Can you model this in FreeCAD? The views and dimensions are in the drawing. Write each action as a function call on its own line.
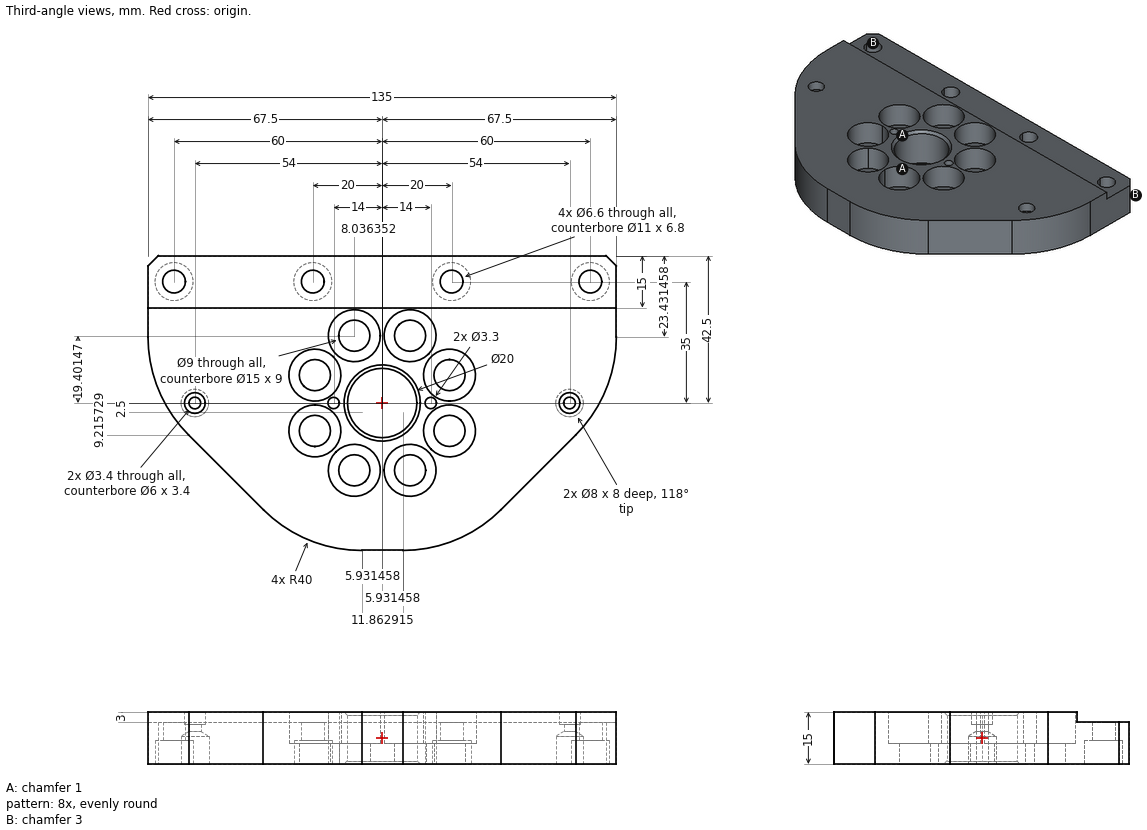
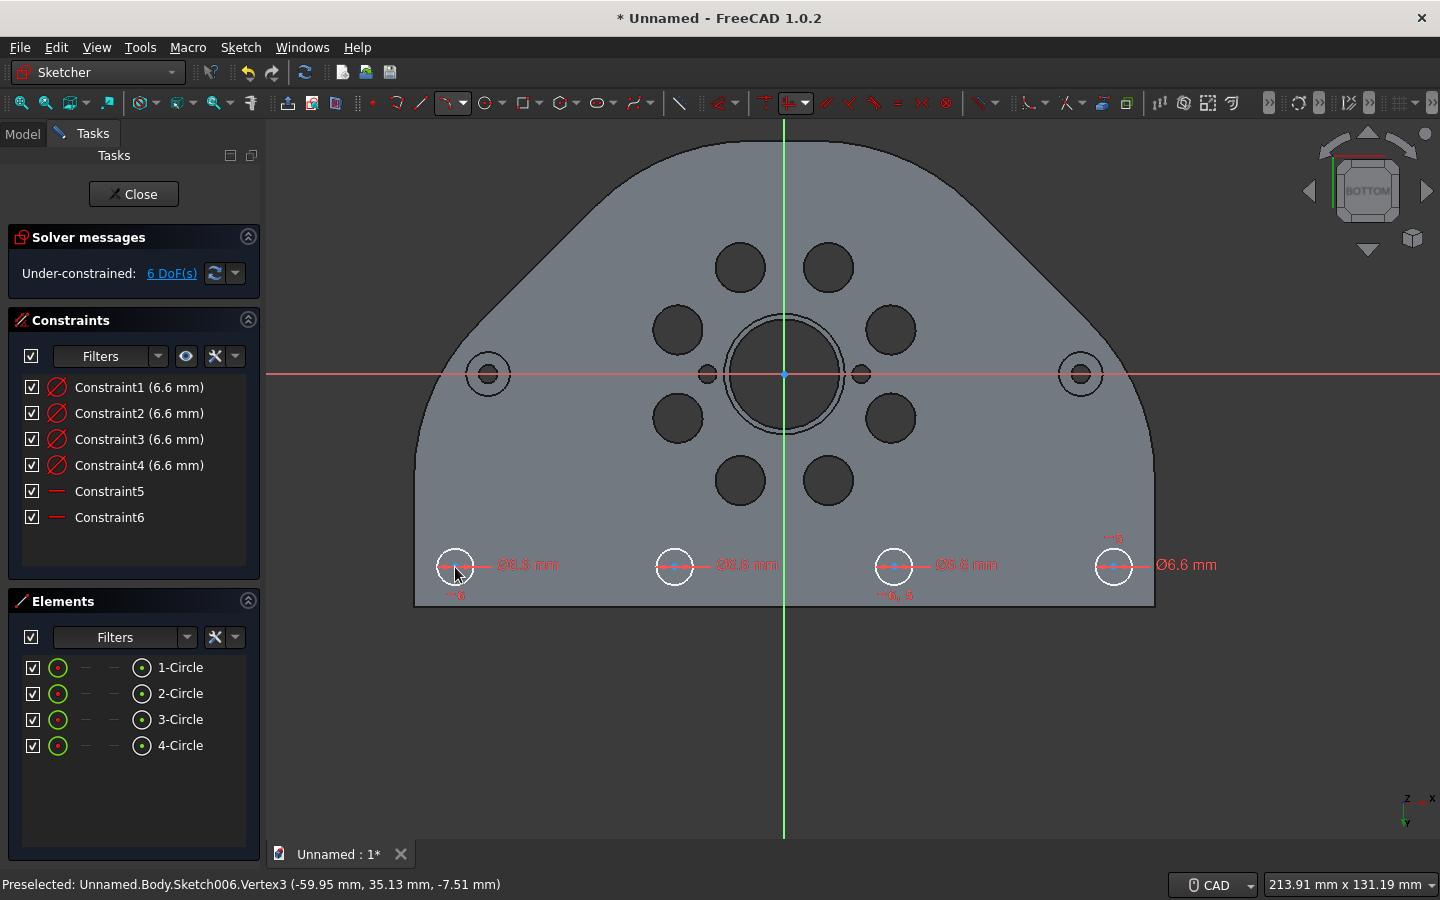
click(894, 567)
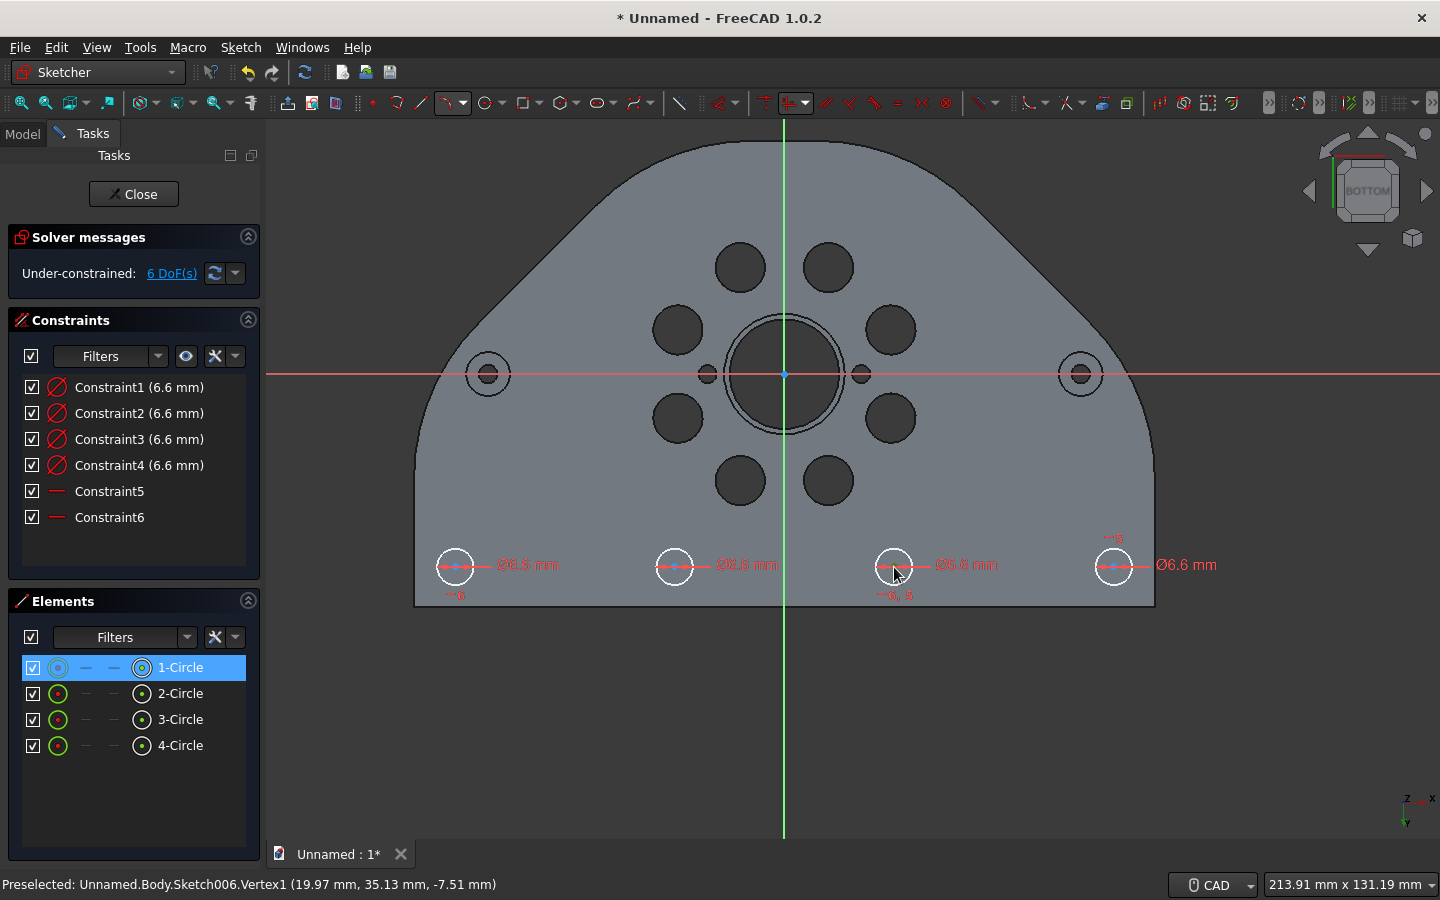
click(675, 567)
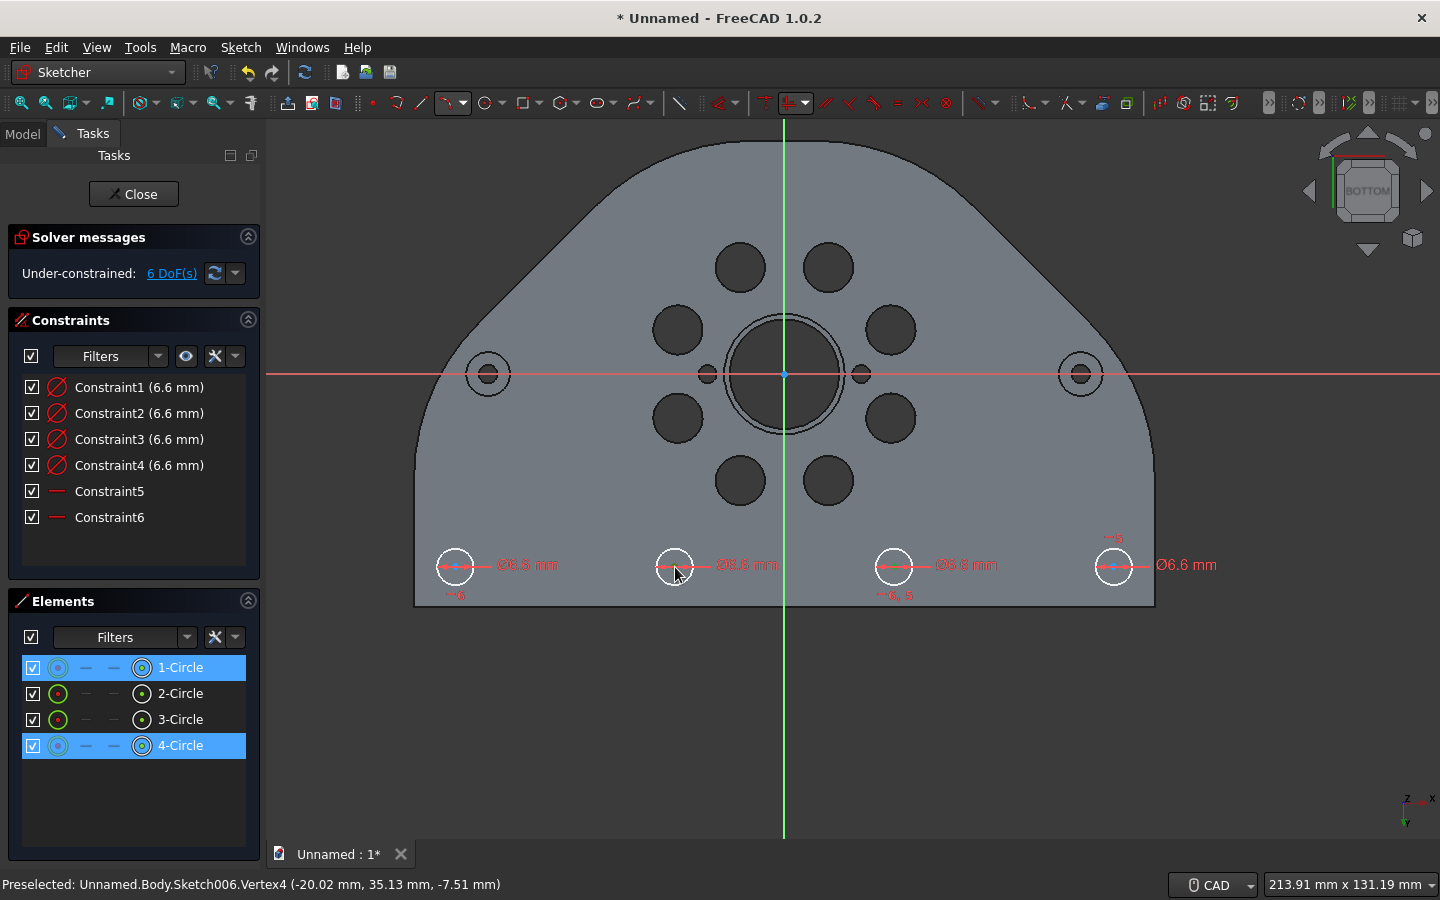
click(808, 104)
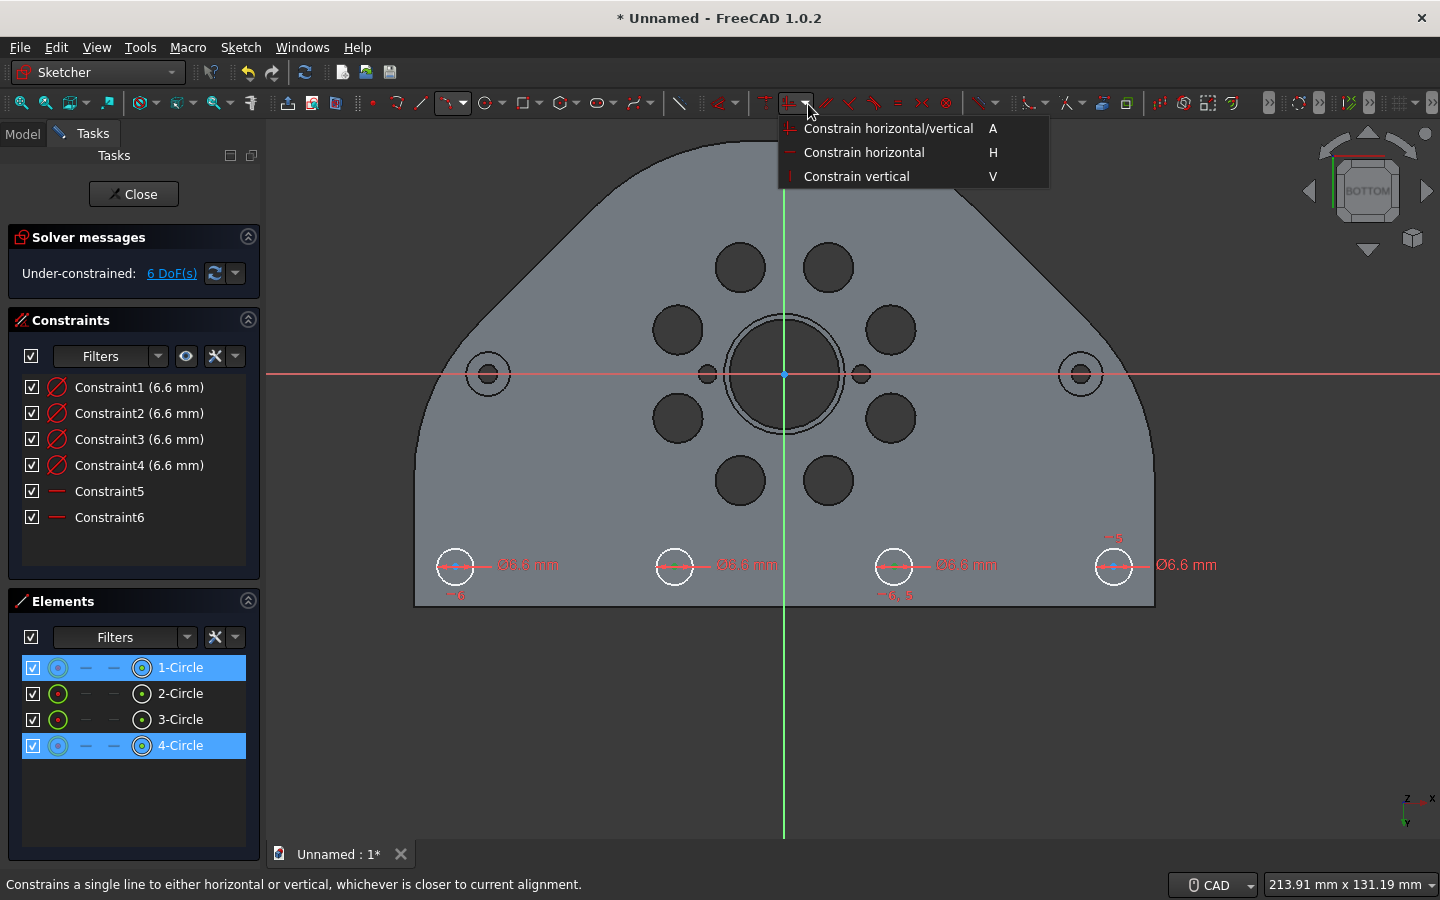
click(914, 152)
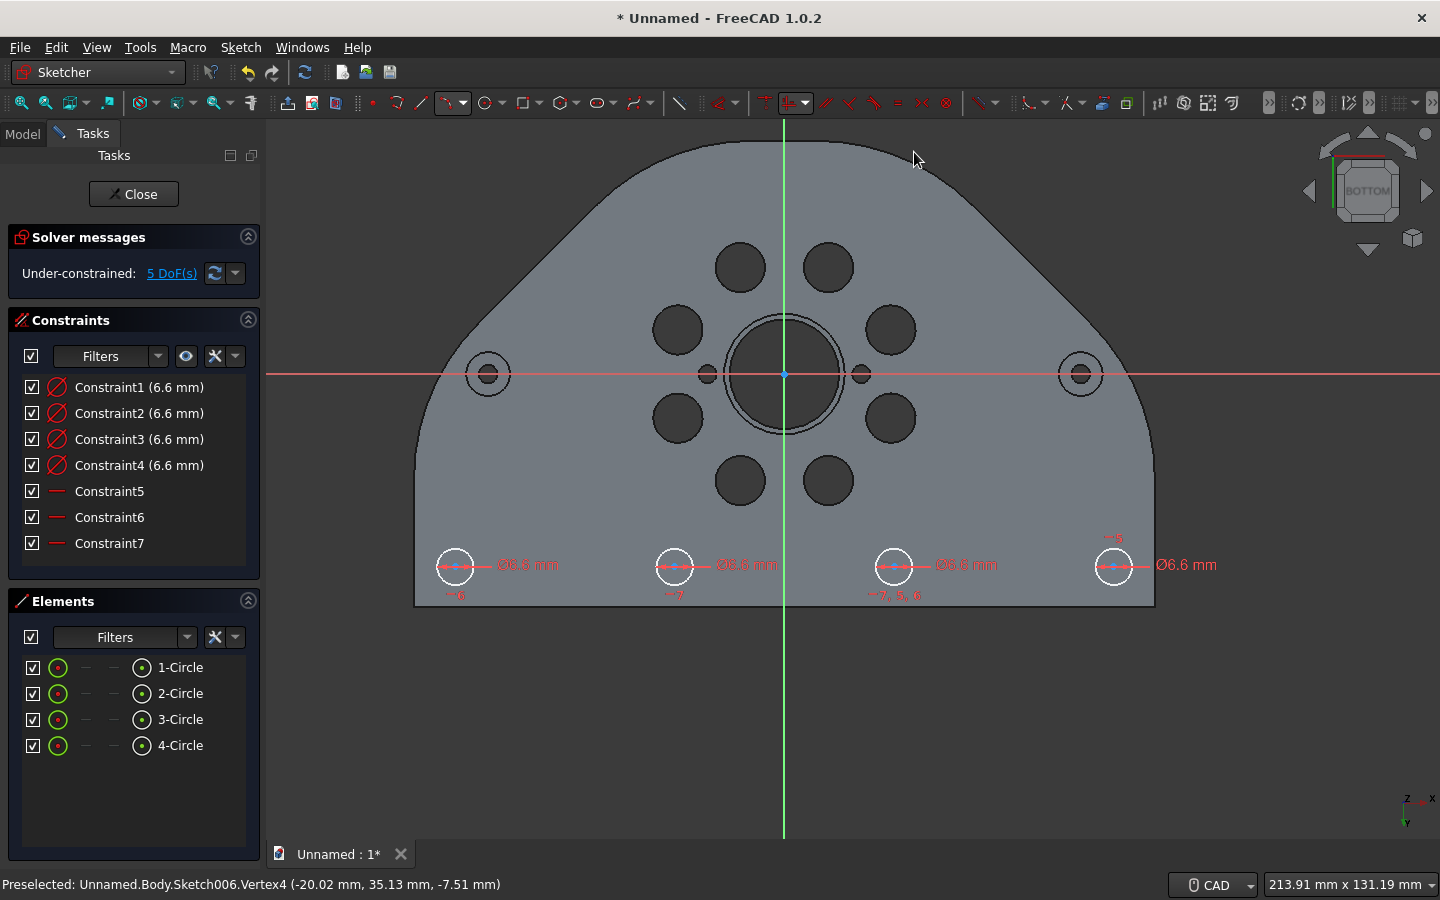
key(d)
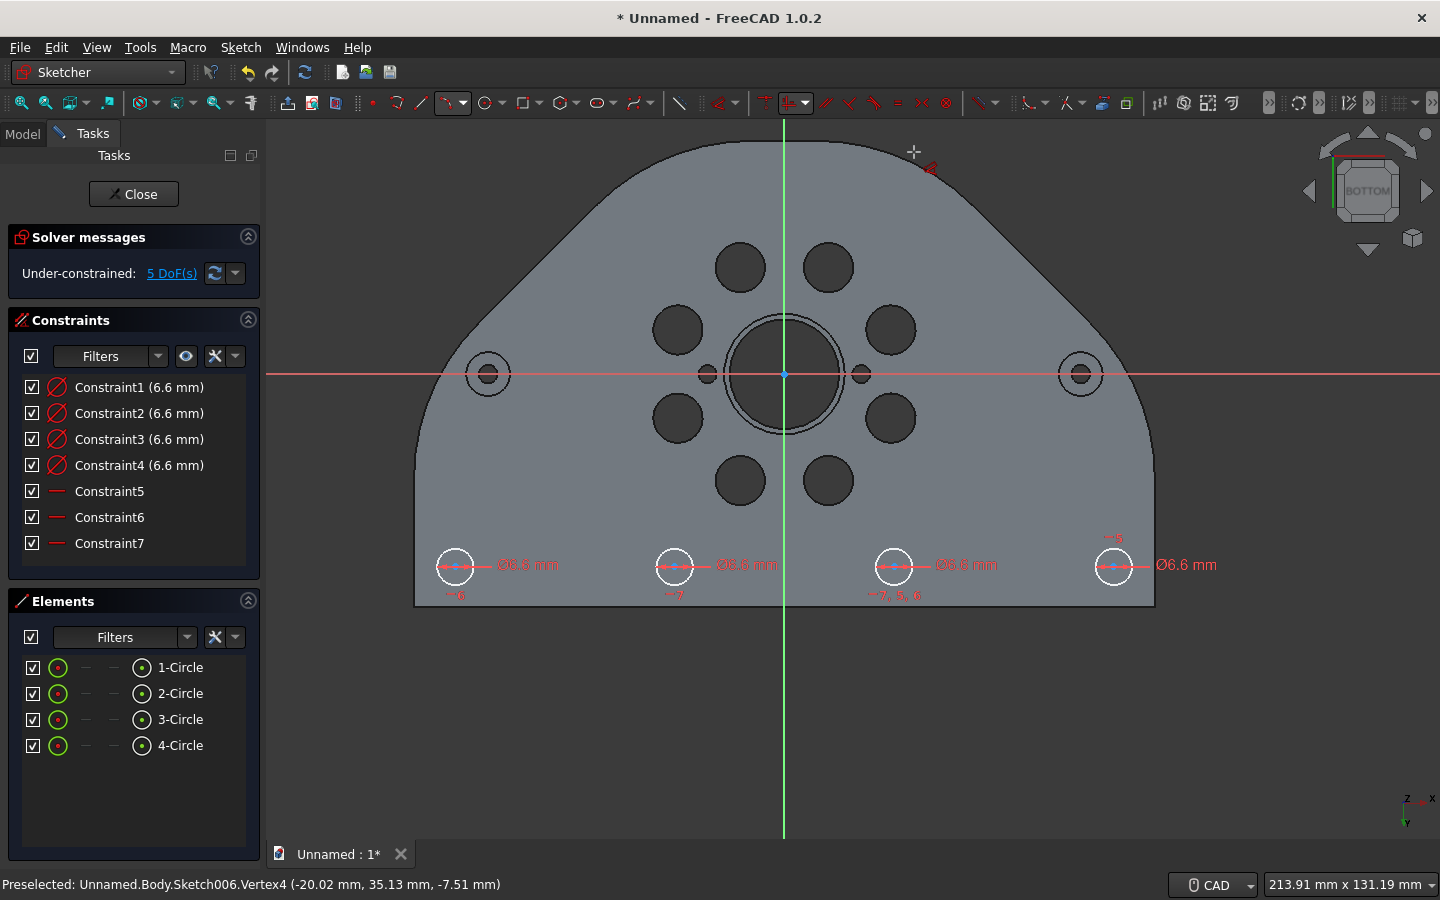
click(894, 567)
click(839, 340)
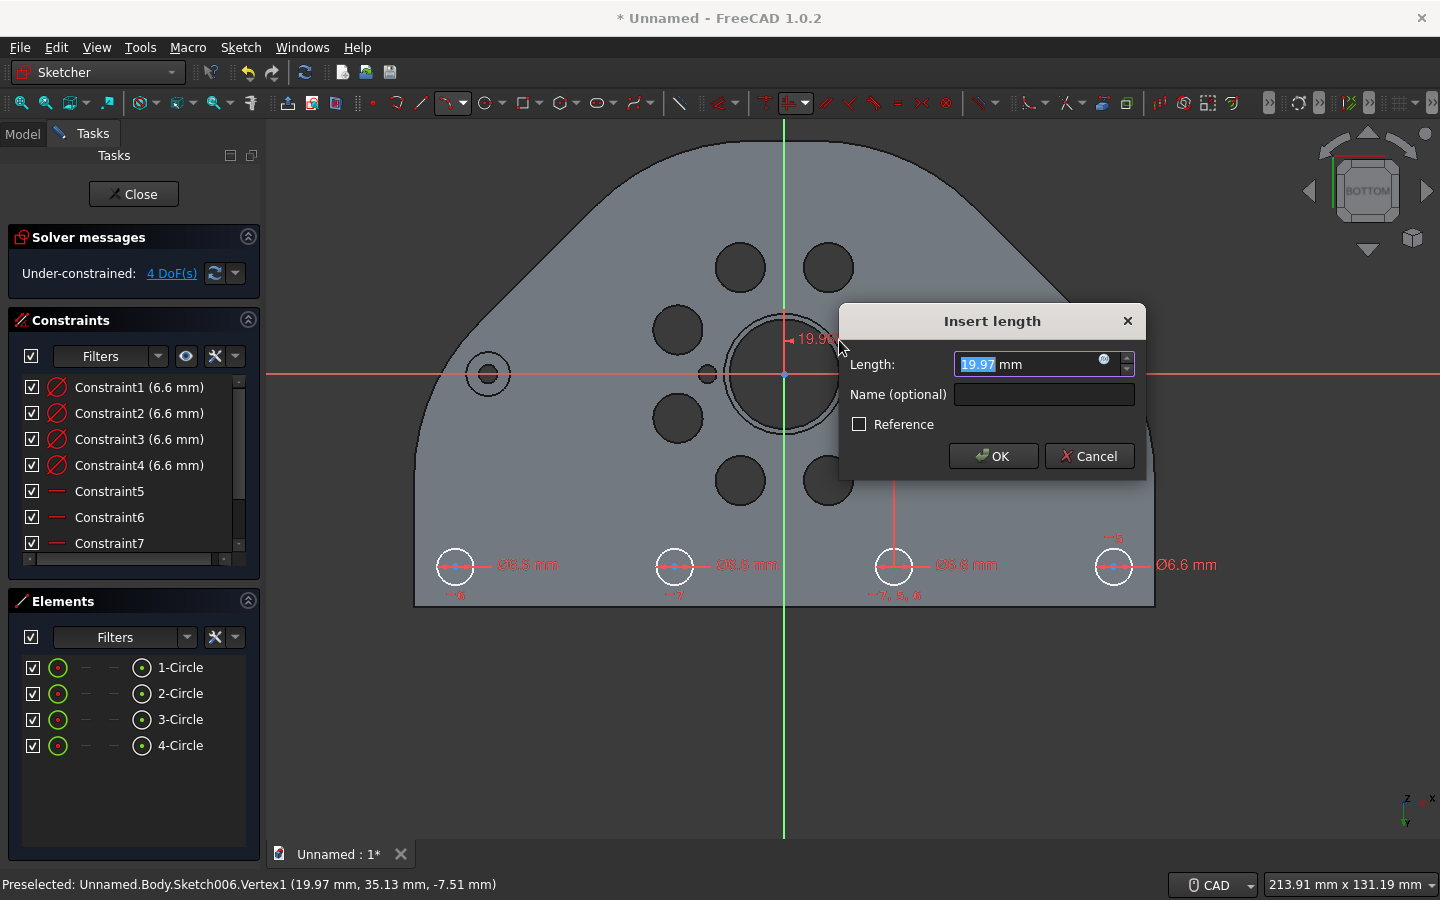
text(20)
key(Return)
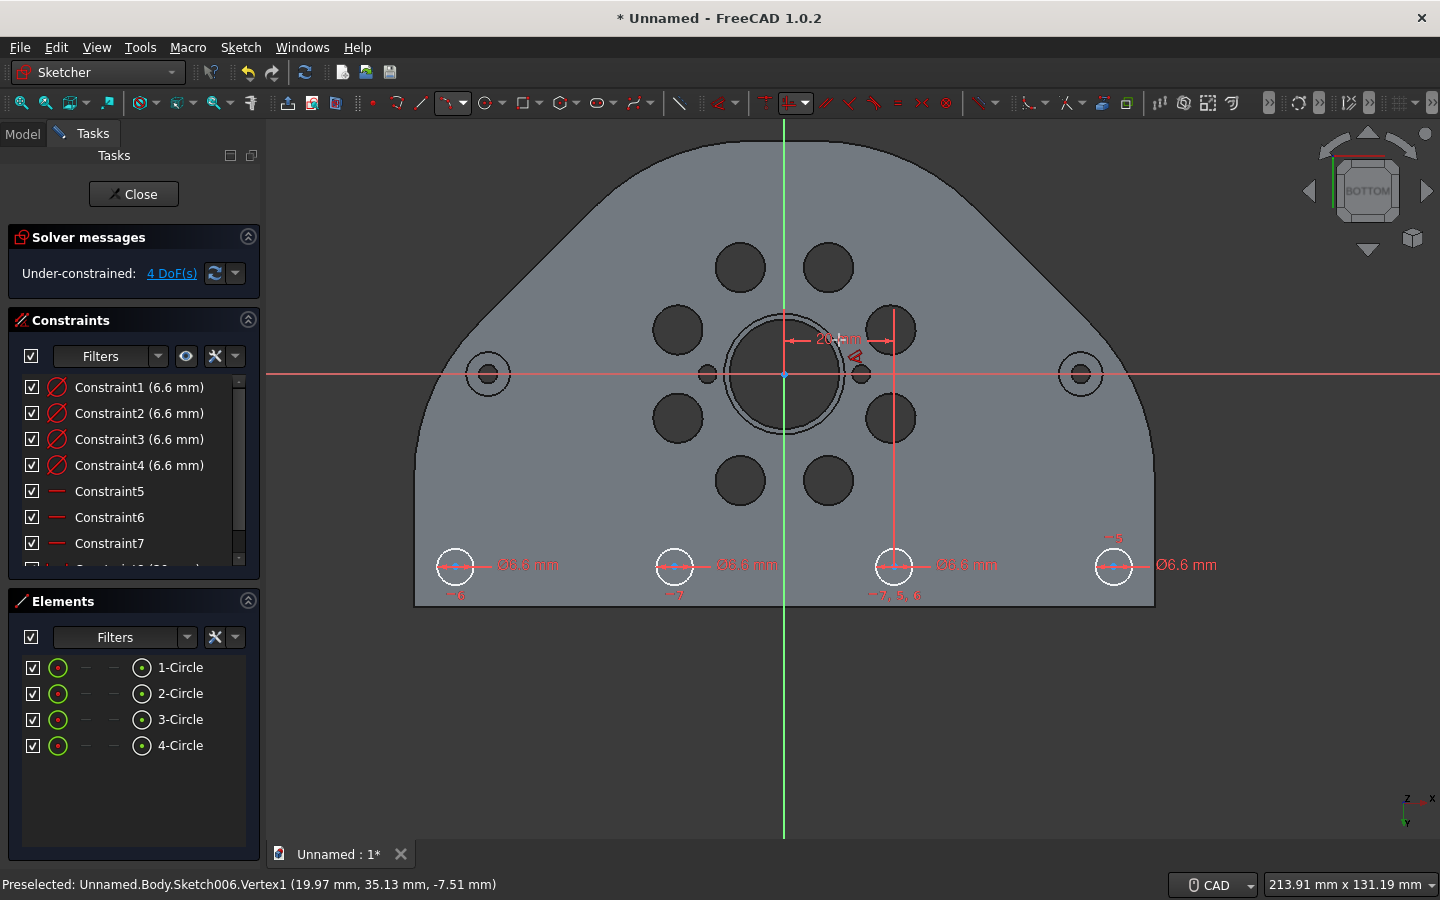
click(894, 567)
click(928, 471)